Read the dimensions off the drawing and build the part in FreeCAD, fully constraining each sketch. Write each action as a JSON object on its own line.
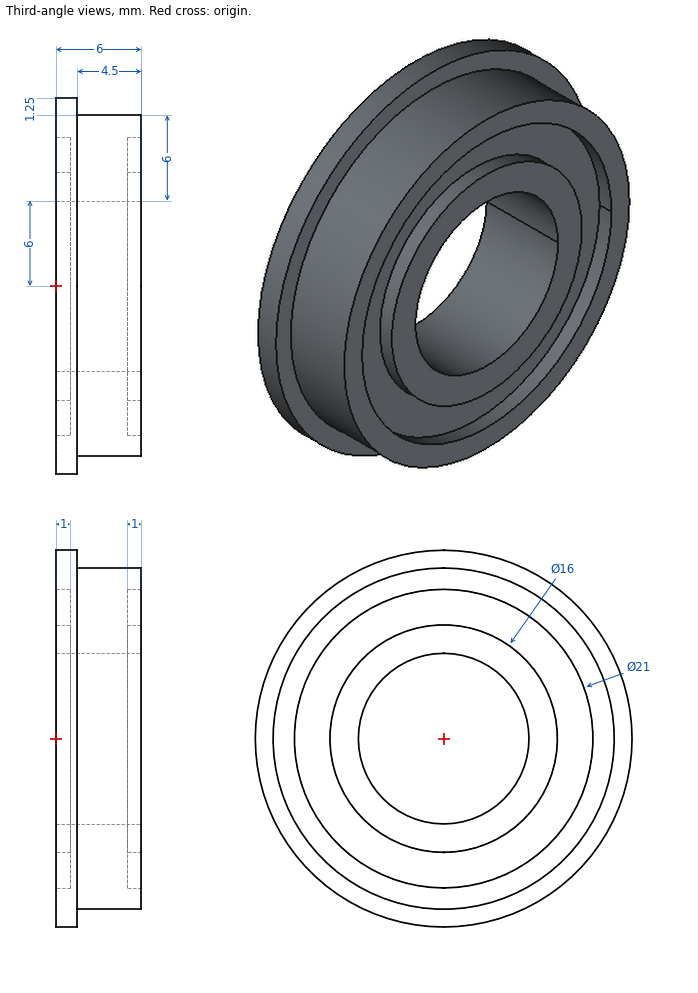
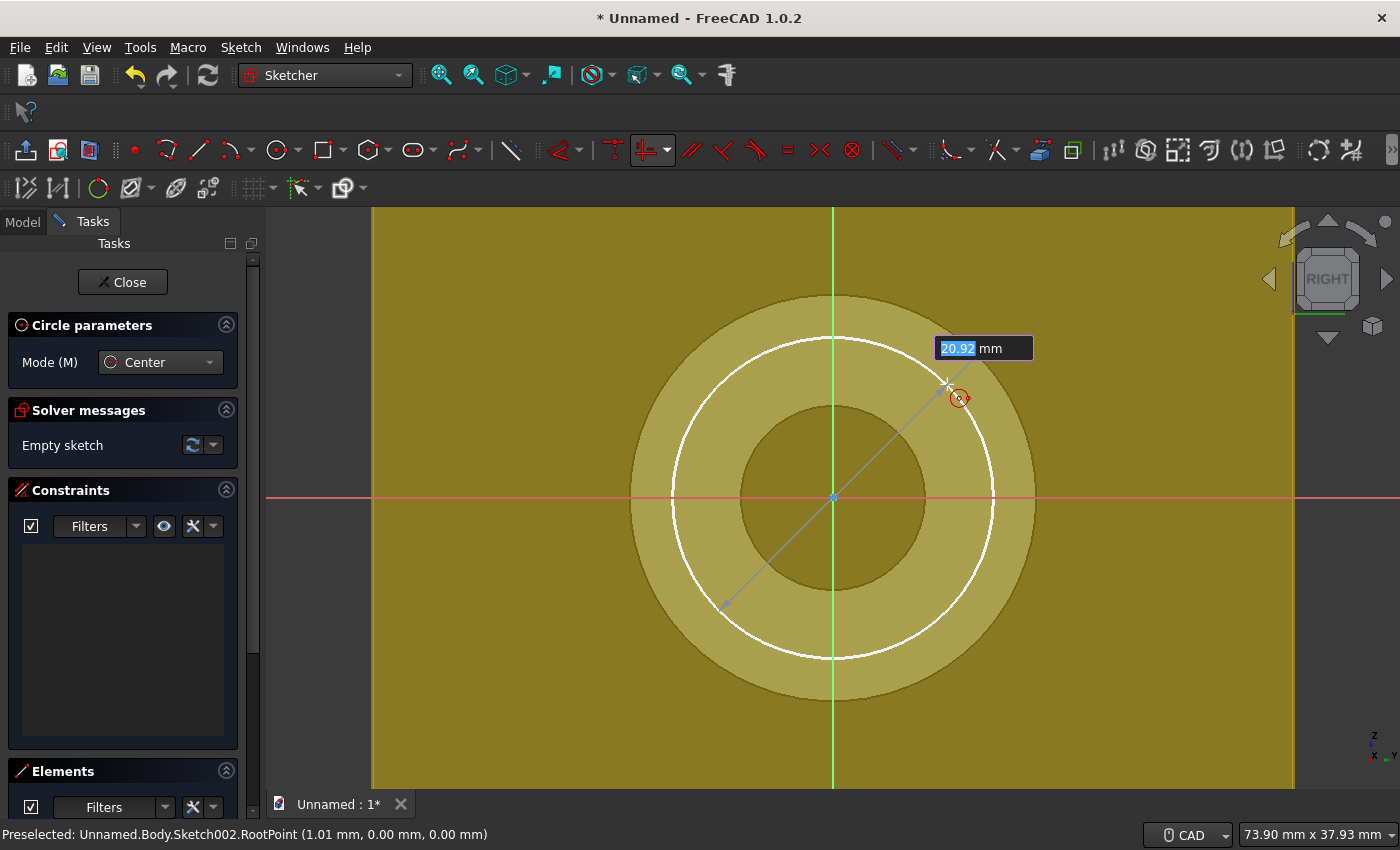
{"action": "type", "text": "21"}
{"action": "key", "text": "Return"}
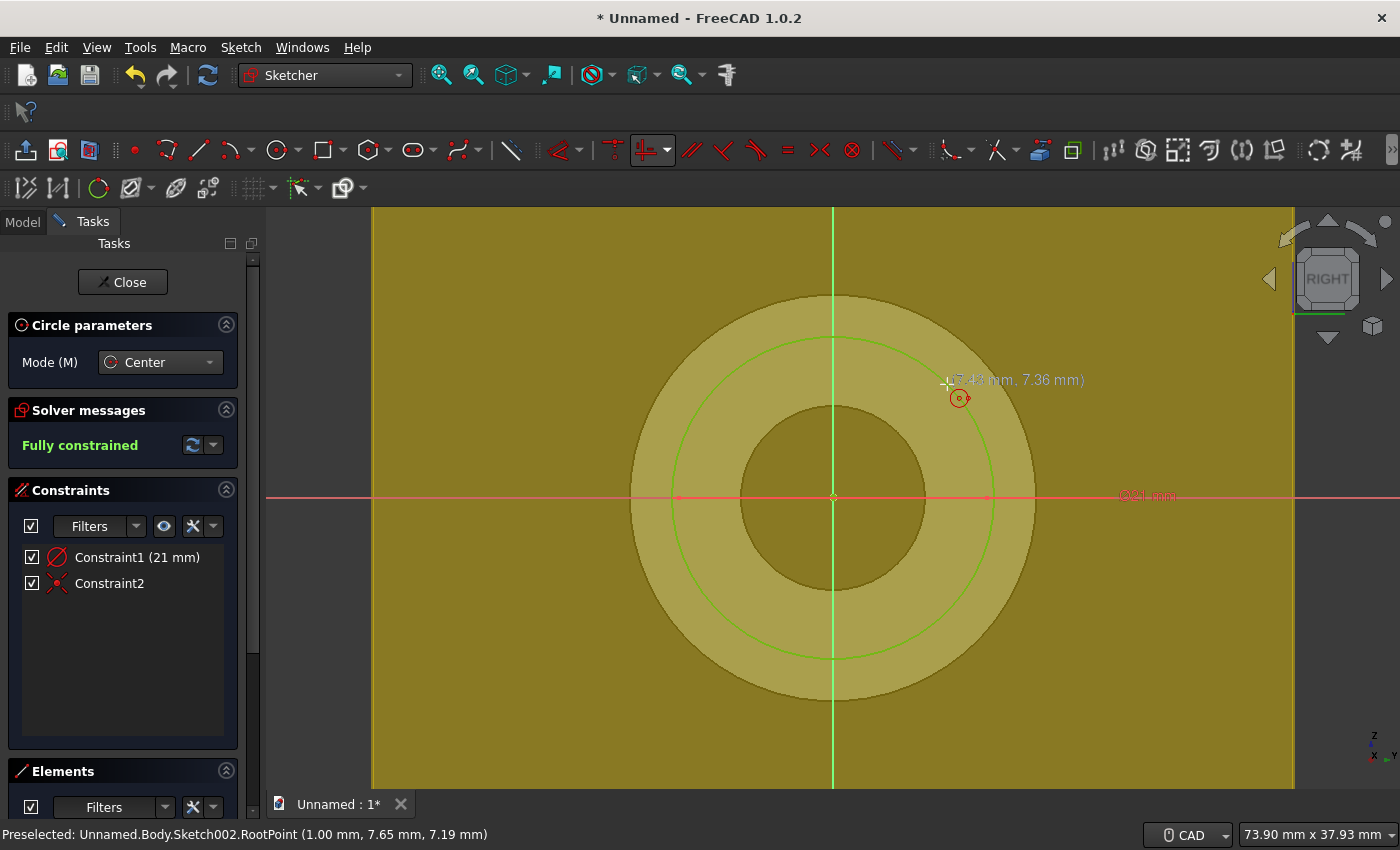
{"action": "left_click", "coordinate": [833, 498]}
{"action": "mouse_move", "coordinate": [920, 411]}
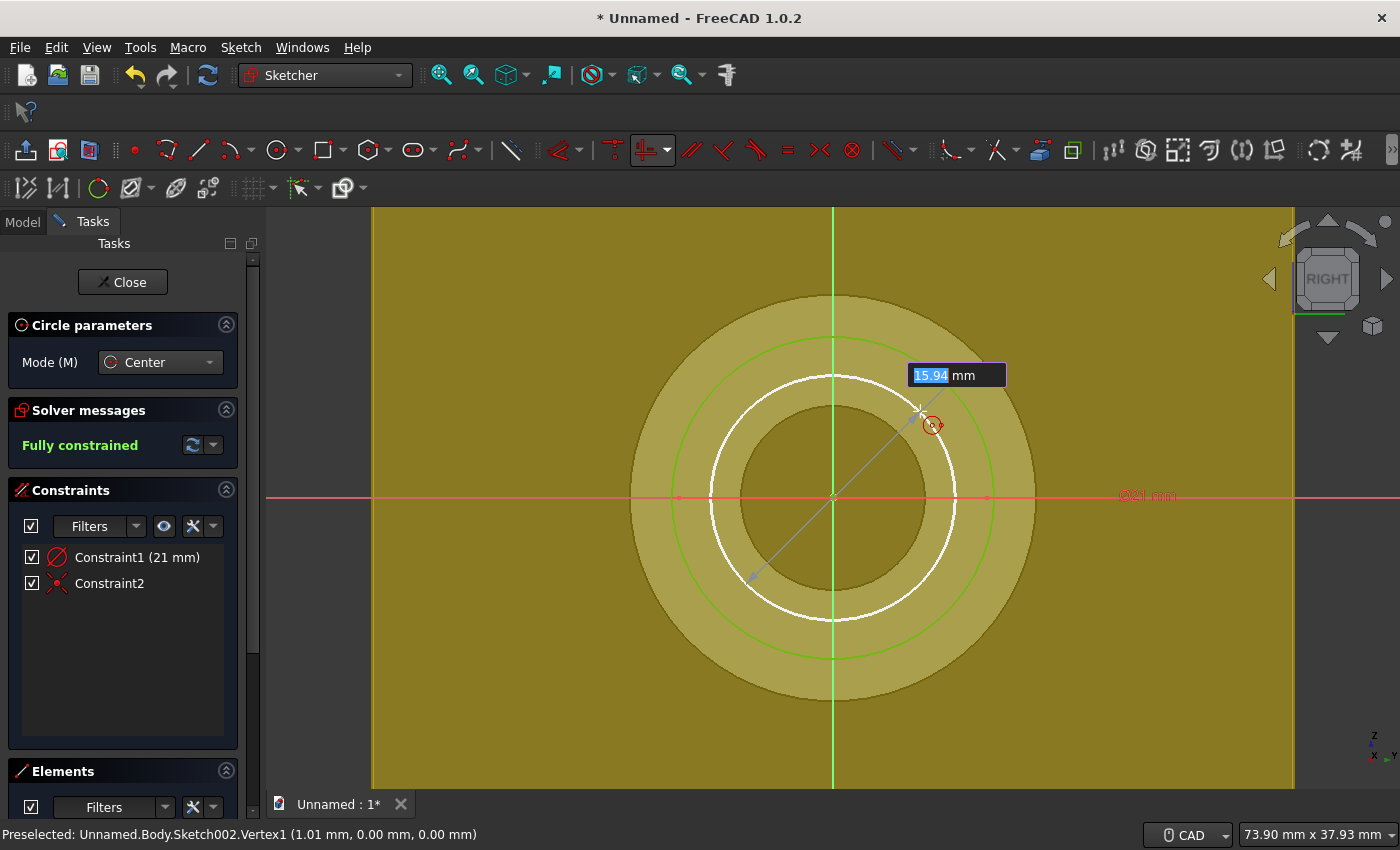
{"action": "type", "text": "16"}
{"action": "key", "text": "Return"}
{"action": "key", "text": "Escape"}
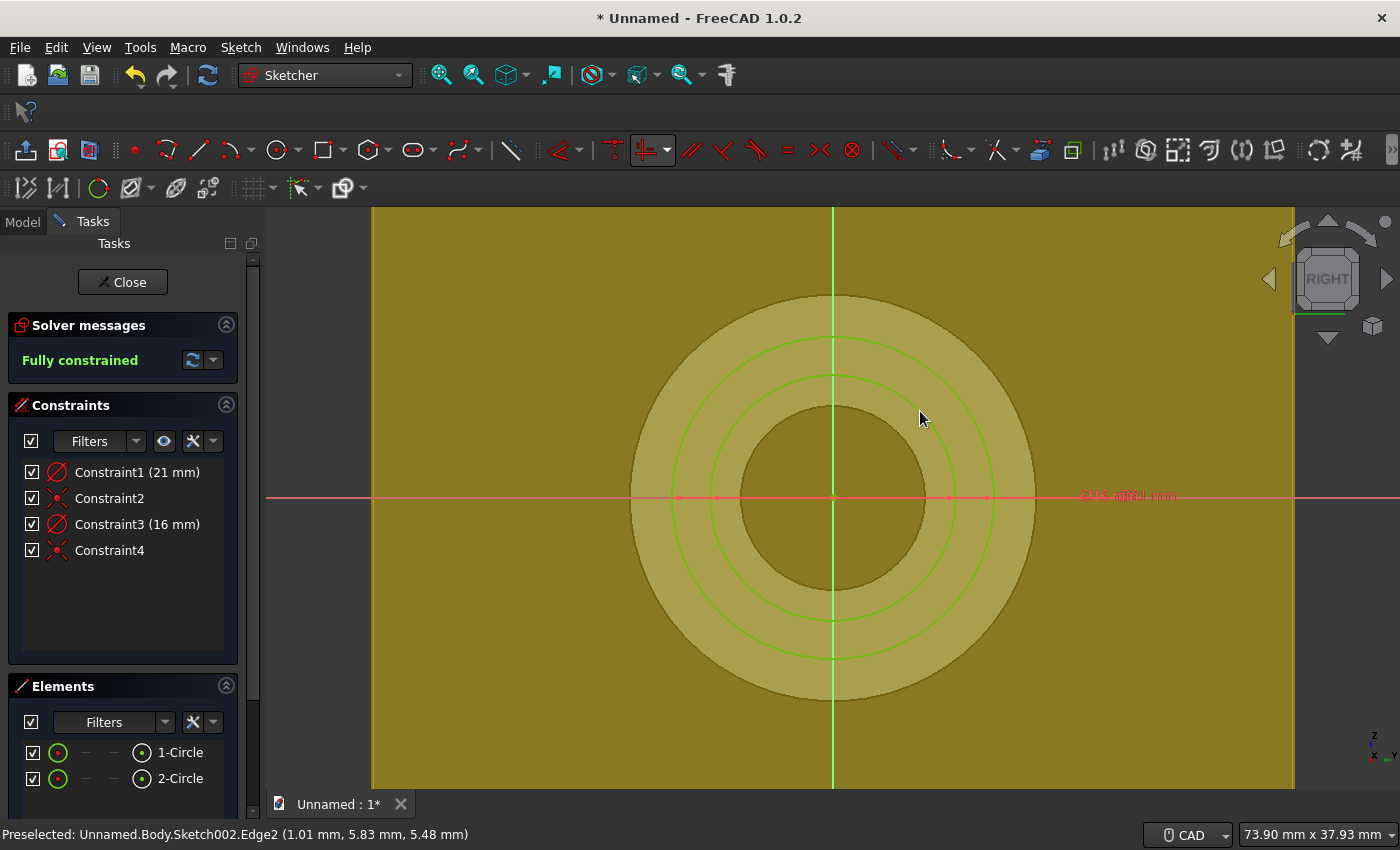
{"action": "left_click", "coordinate": [123, 282]}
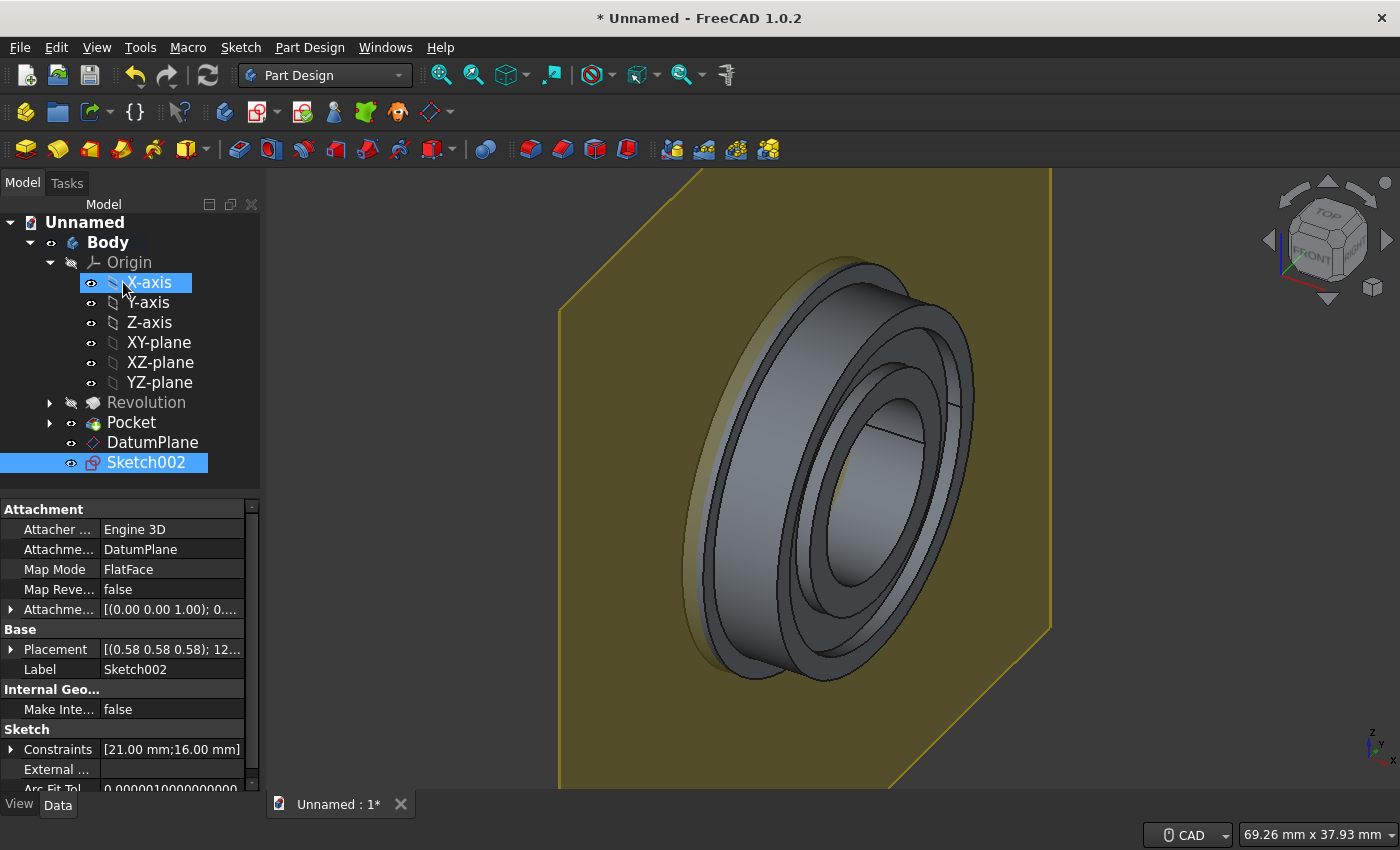
{"action": "left_click", "coordinate": [240, 150]}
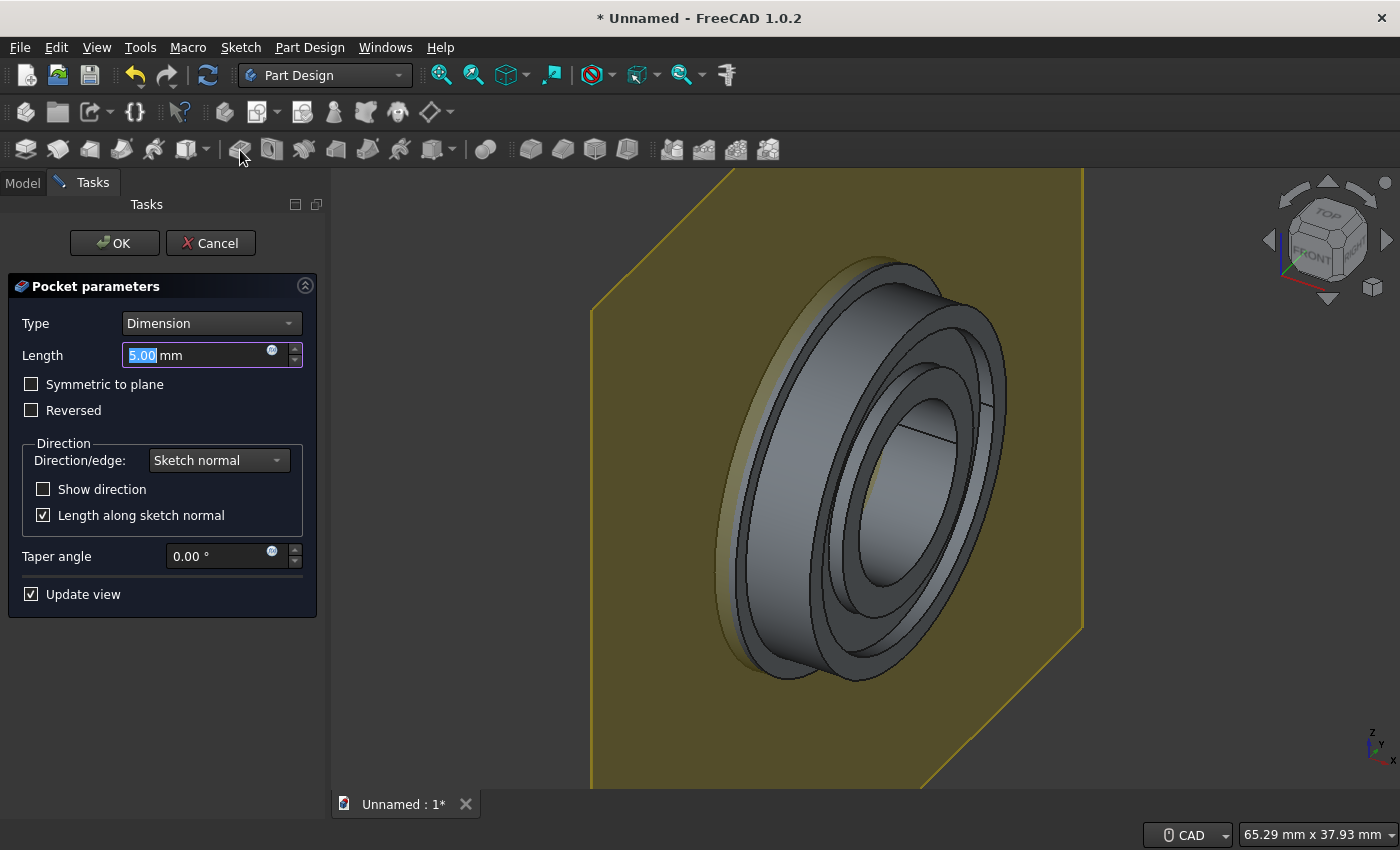
{"action": "type", "text": "1"}
{"action": "key", "text": "Tab"}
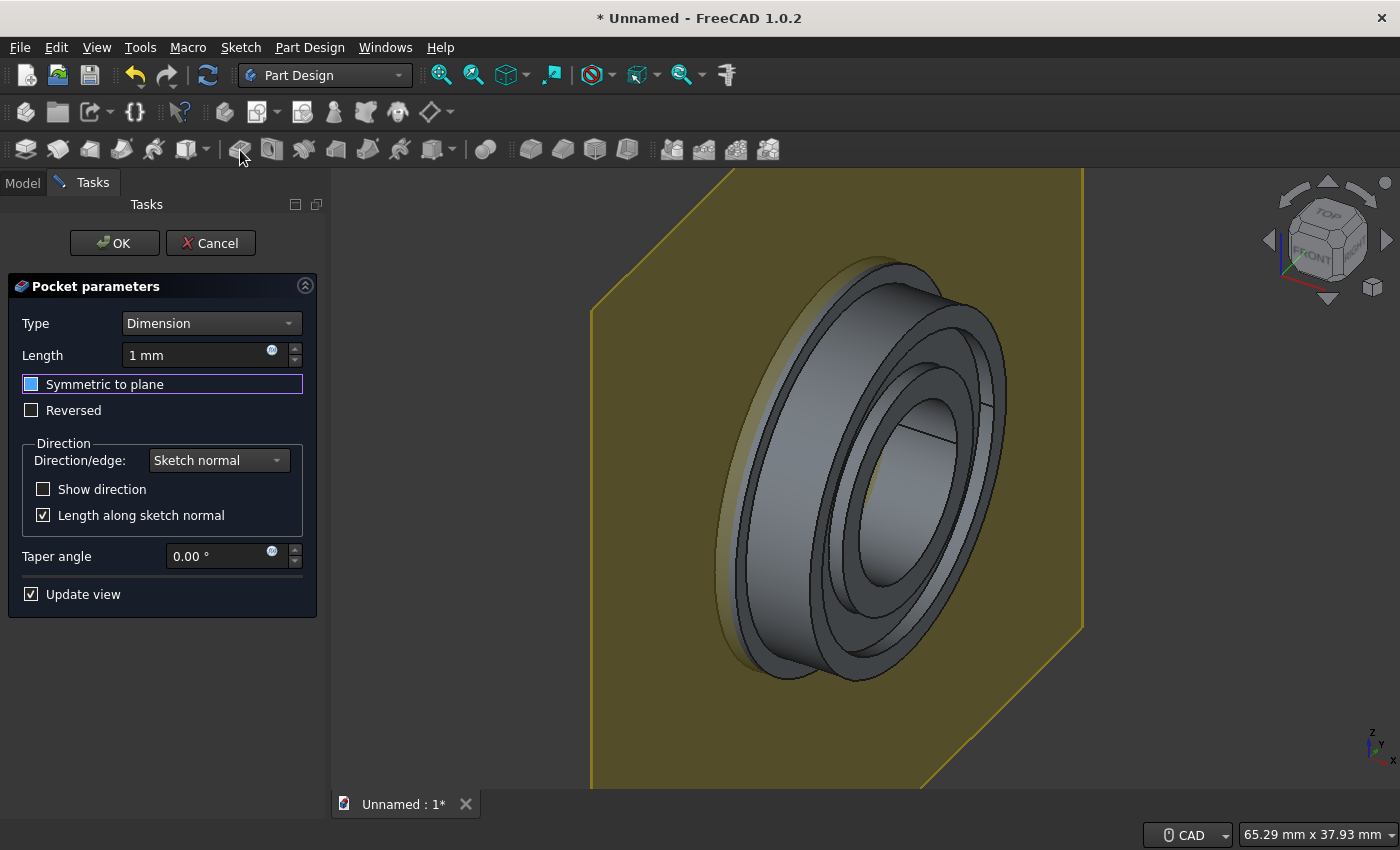
{"action": "left_click", "coordinate": [115, 243]}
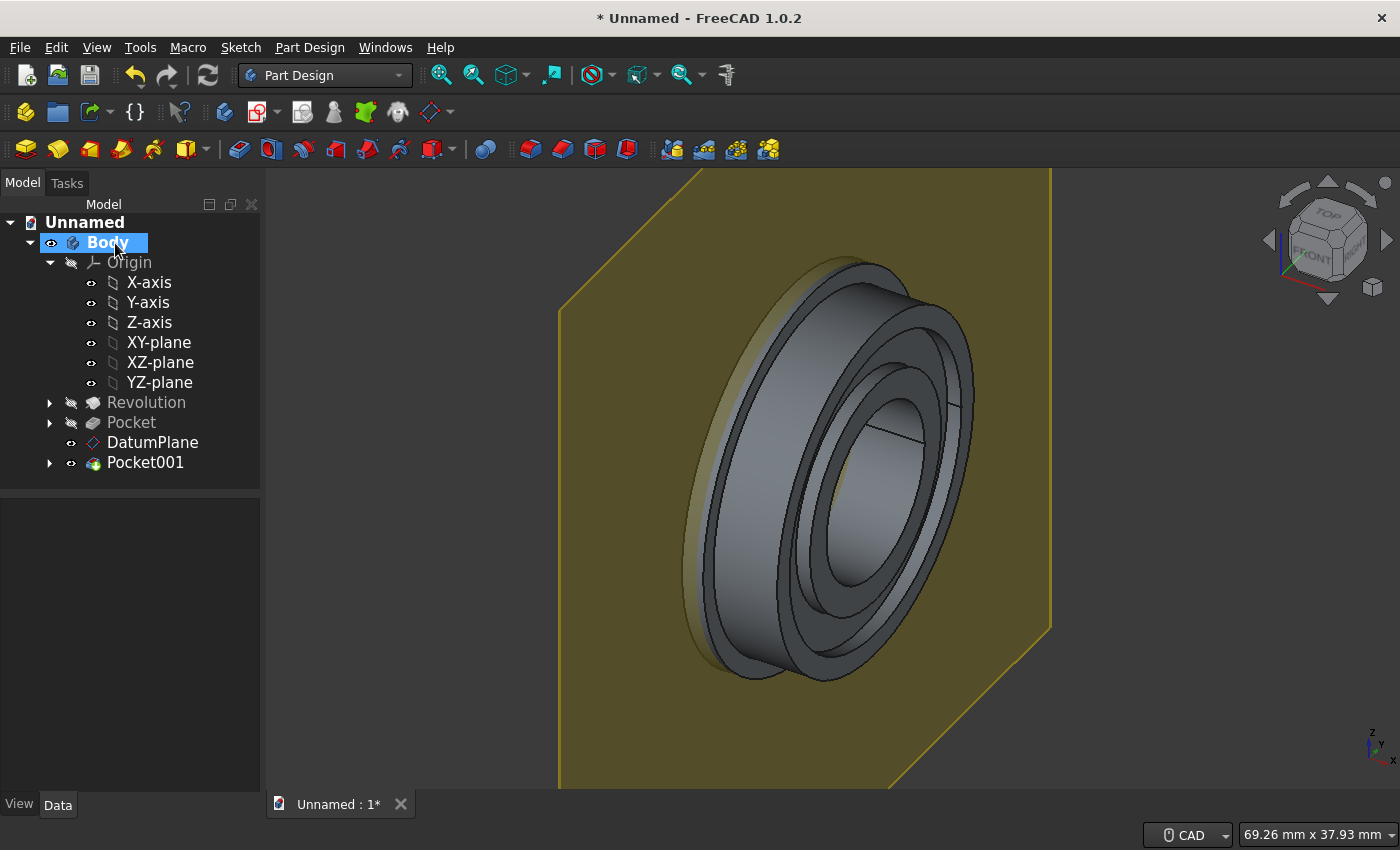
{"action": "left_click", "coordinate": [116, 443]}
{"action": "key", "text": "space"}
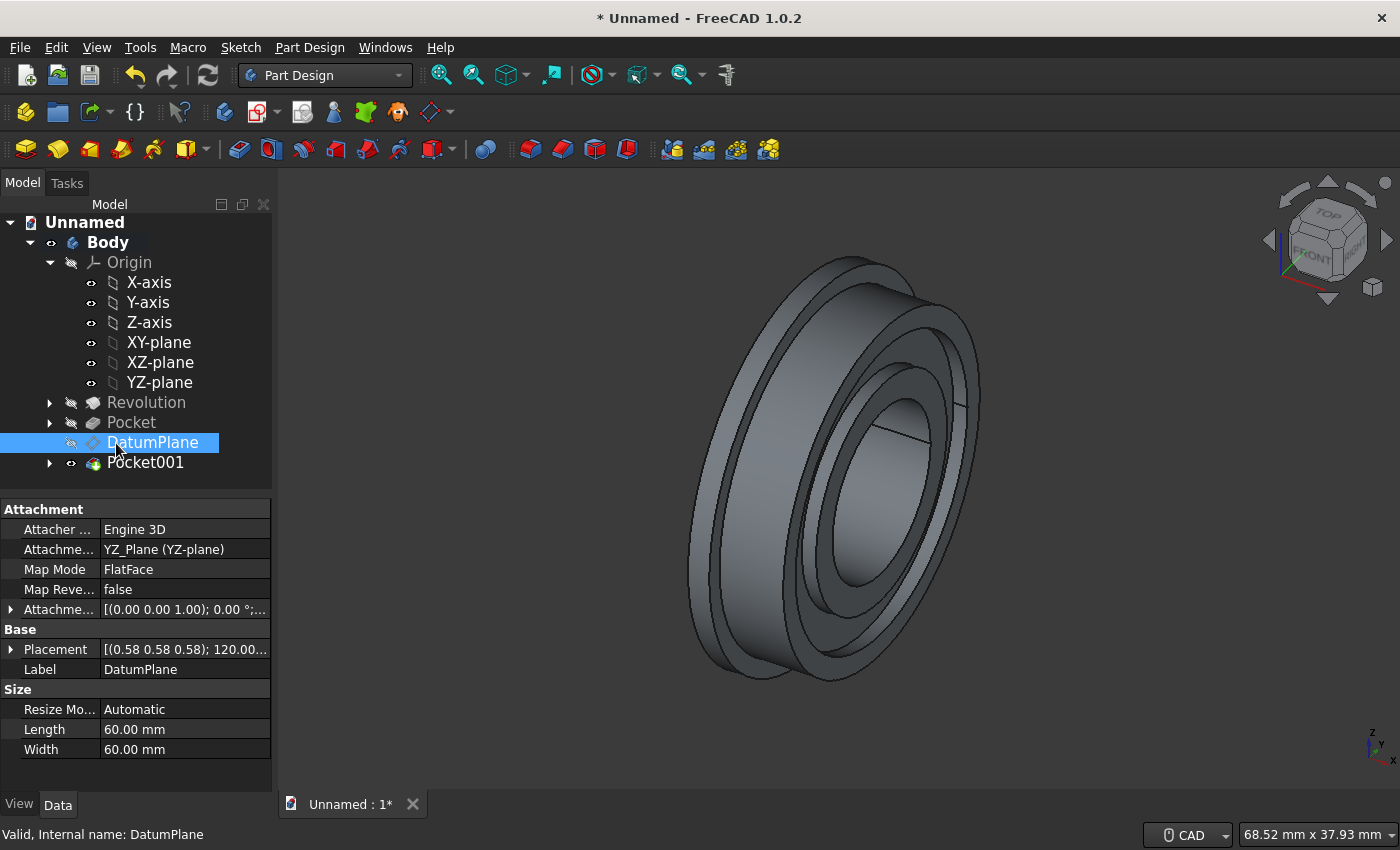
{"action": "key", "text": "0"}